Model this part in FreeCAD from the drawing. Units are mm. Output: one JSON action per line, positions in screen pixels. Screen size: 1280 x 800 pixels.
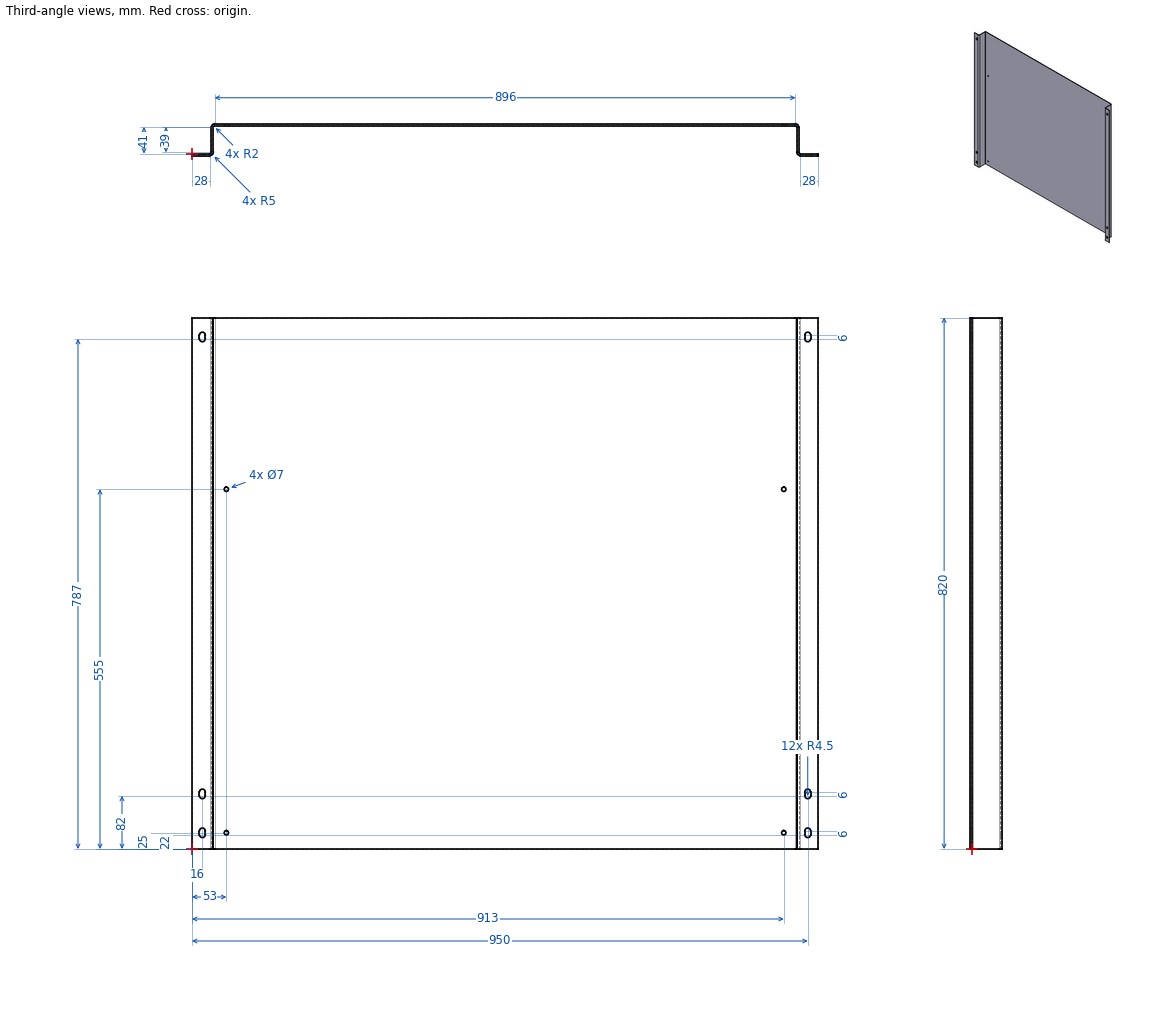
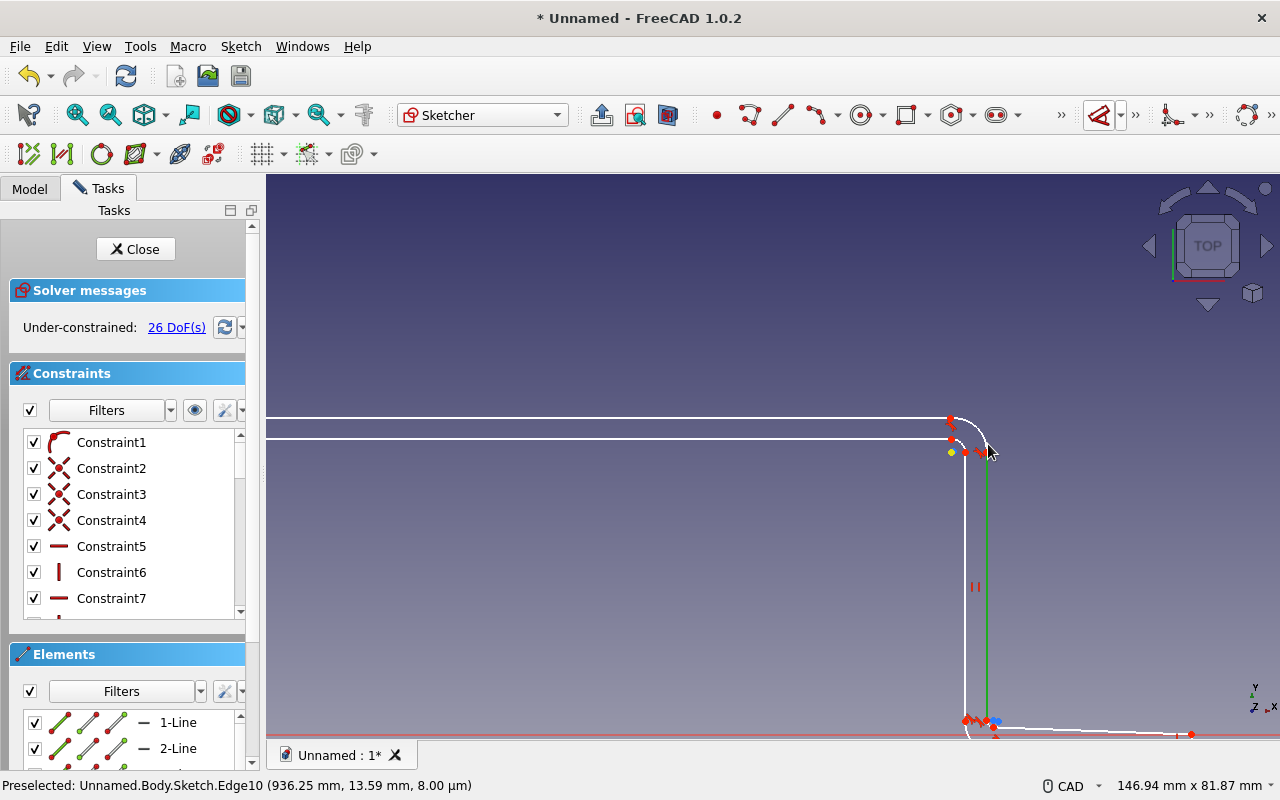
{"action": "left_click", "coordinate": [983, 436]}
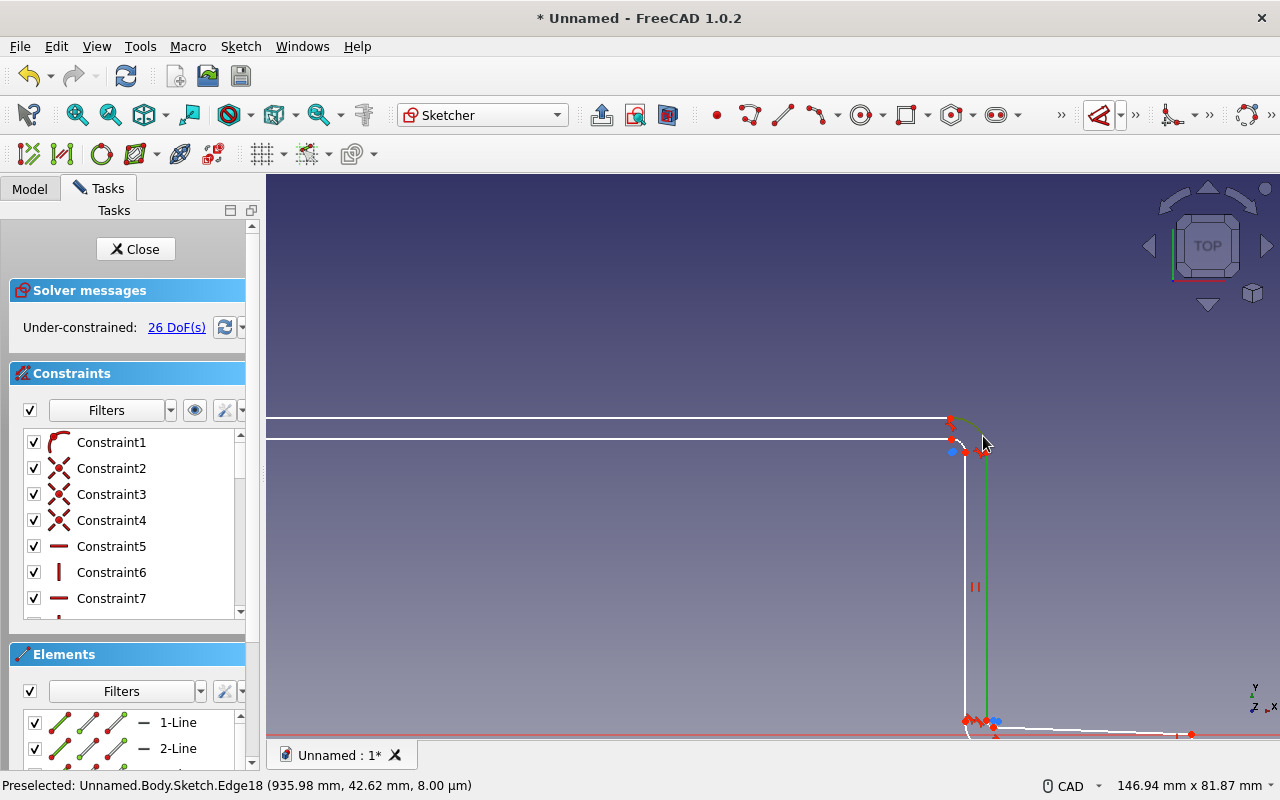
{"action": "key", "text": "t"}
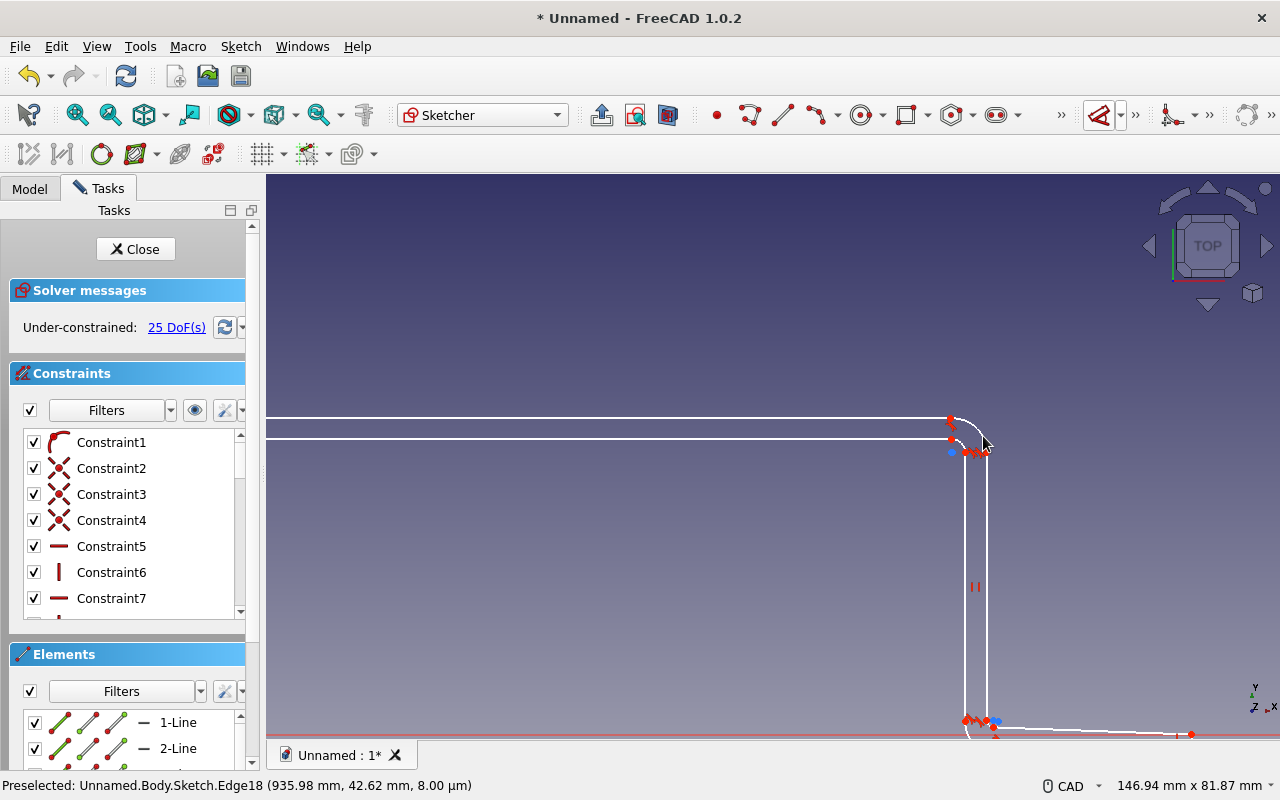
{"action": "scroll", "coordinate": [988, 444], "scroll_direction": "down", "scroll_amount": 12}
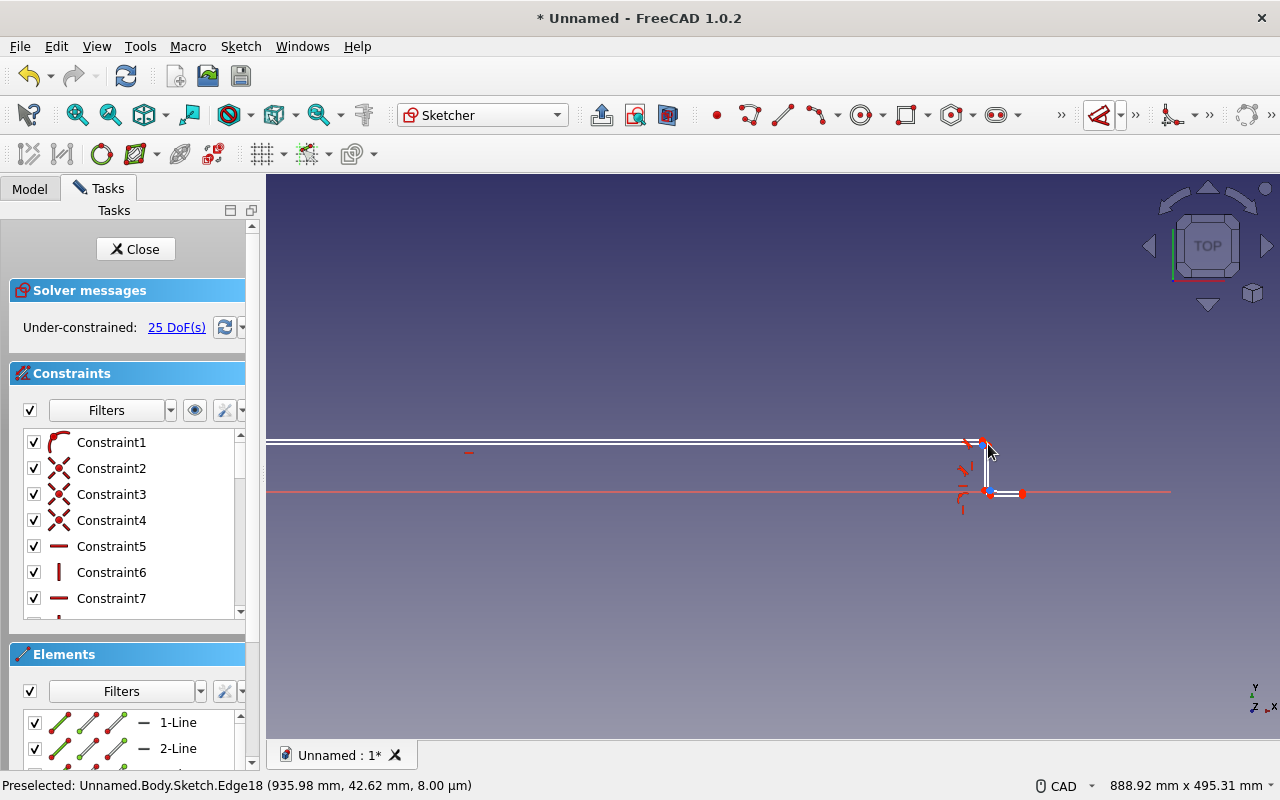
{"action": "scroll", "coordinate": [817, 442], "scroll_direction": "up", "scroll_amount": 10}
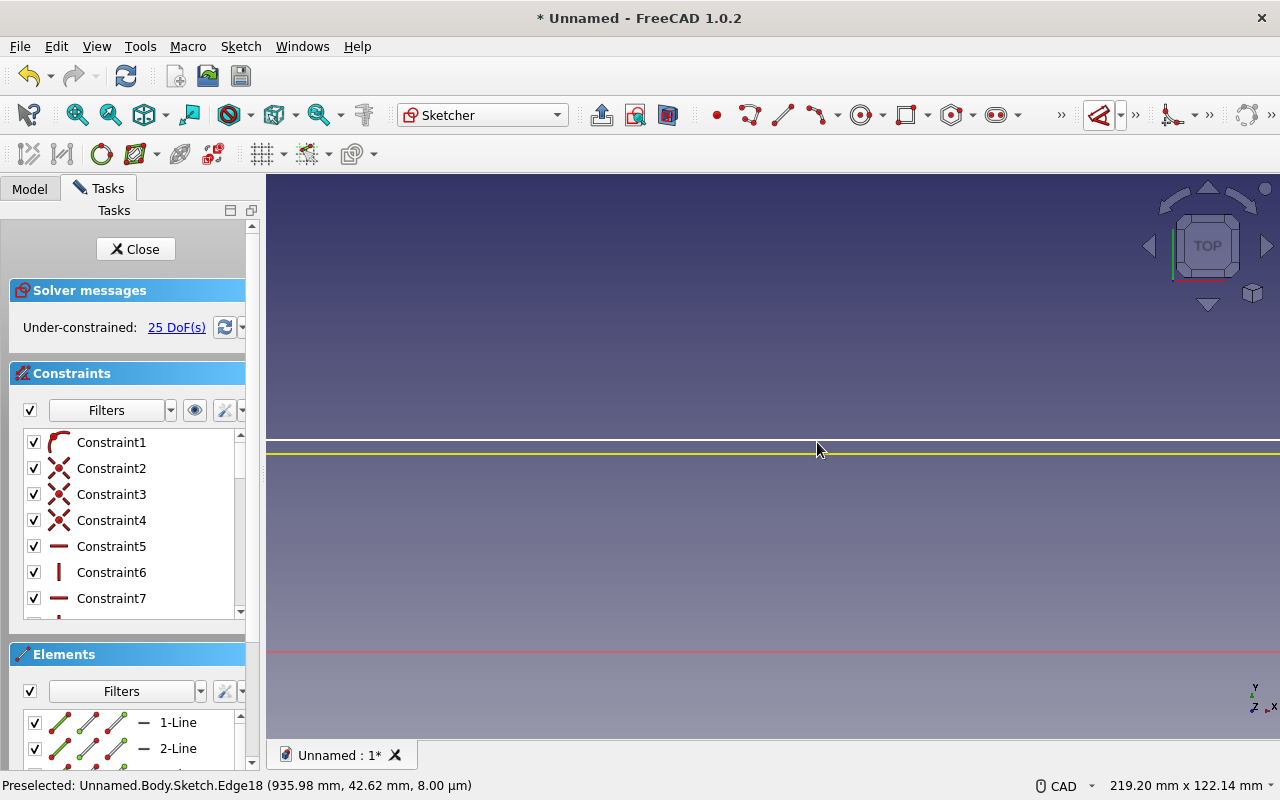
{"action": "left_click", "coordinate": [813, 440]}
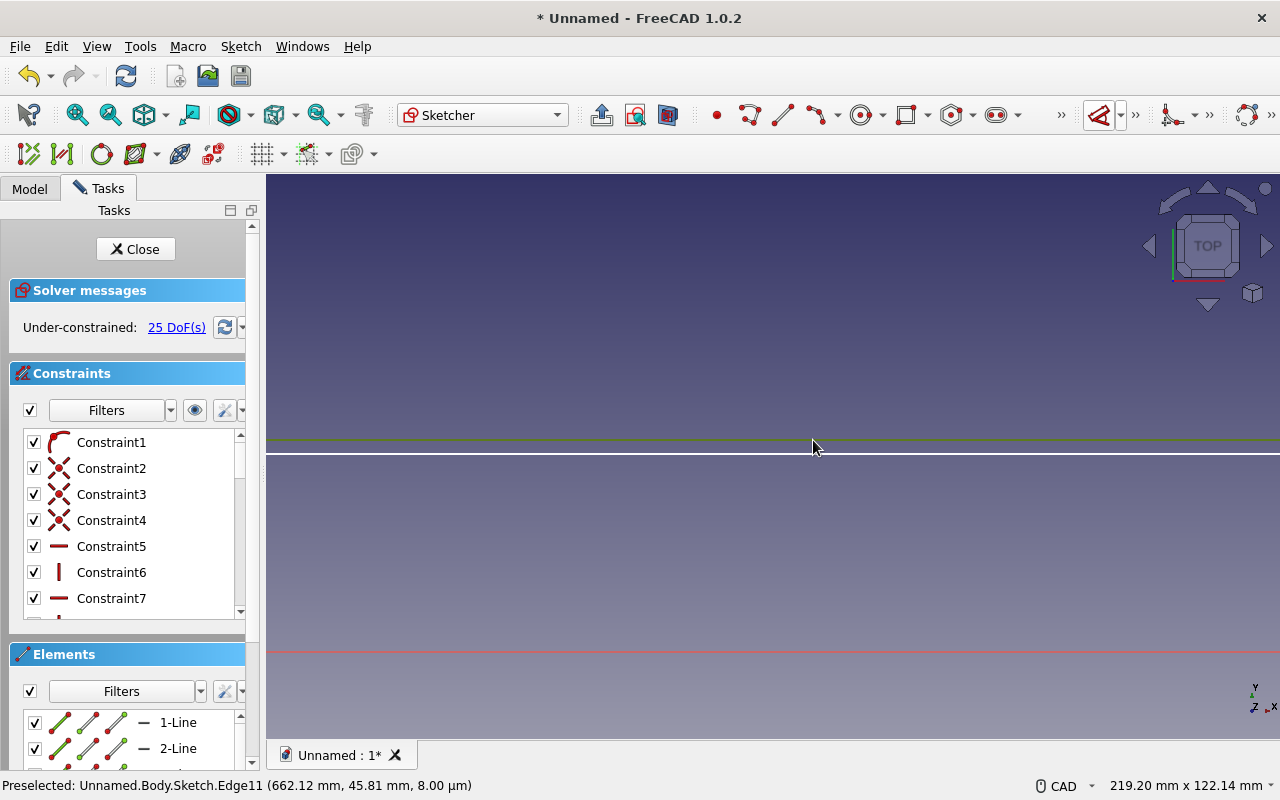
{"action": "scroll", "coordinate": [817, 442], "scroll_direction": "down", "scroll_amount": 10}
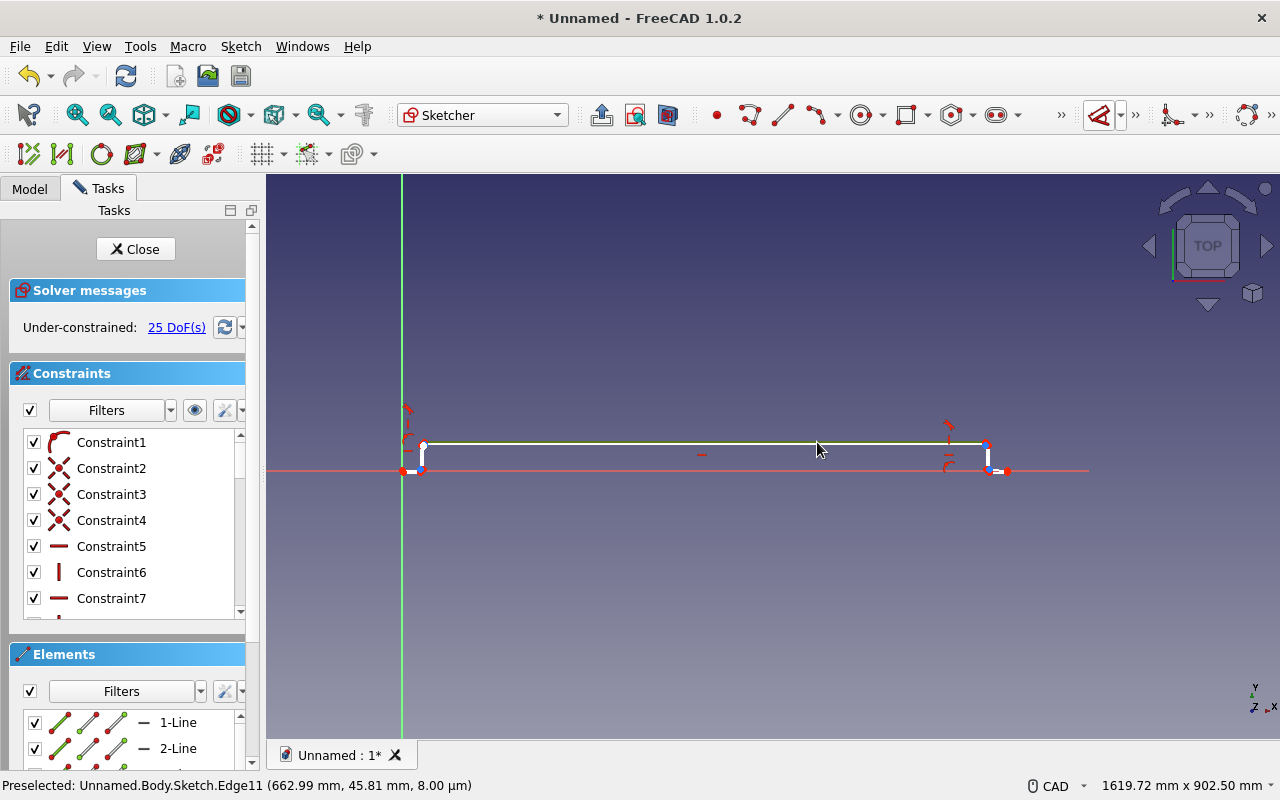
{"action": "scroll", "coordinate": [988, 444], "scroll_direction": "up", "scroll_amount": 12}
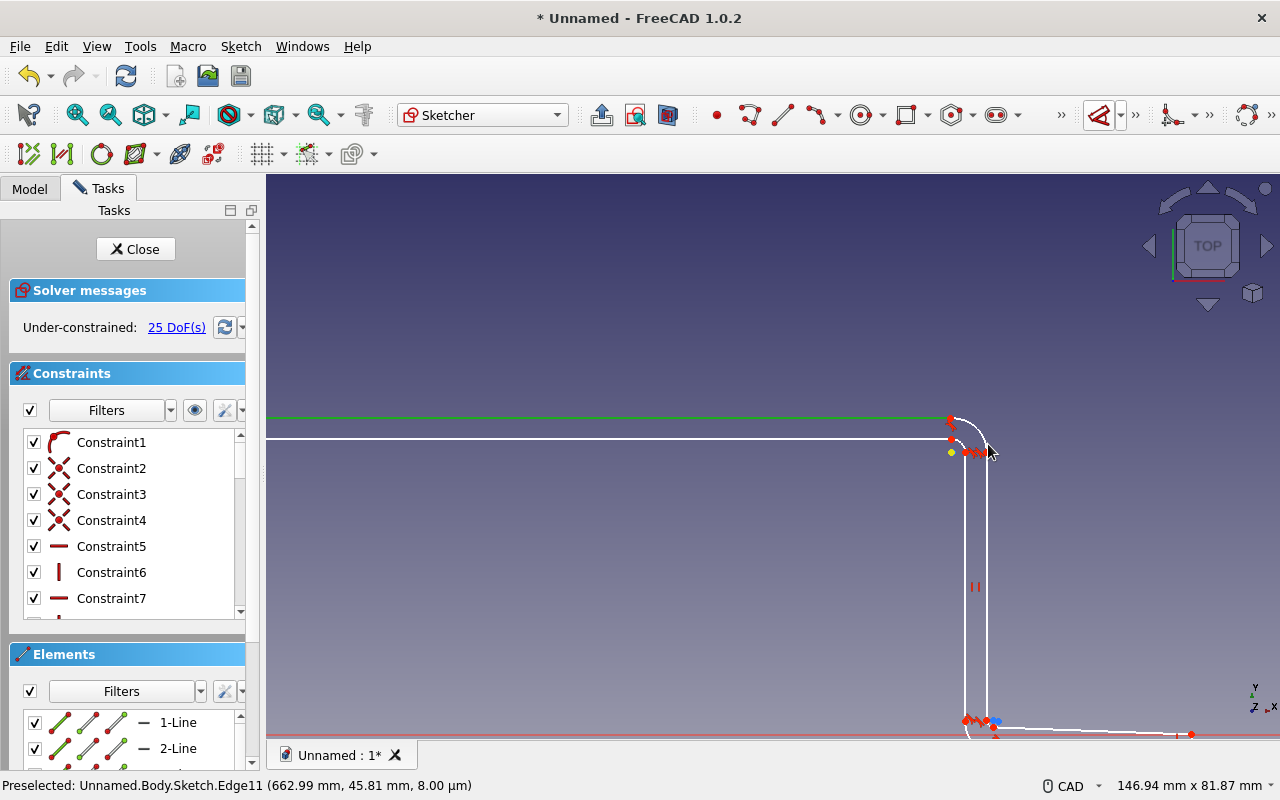
{"action": "left_click", "coordinate": [983, 436]}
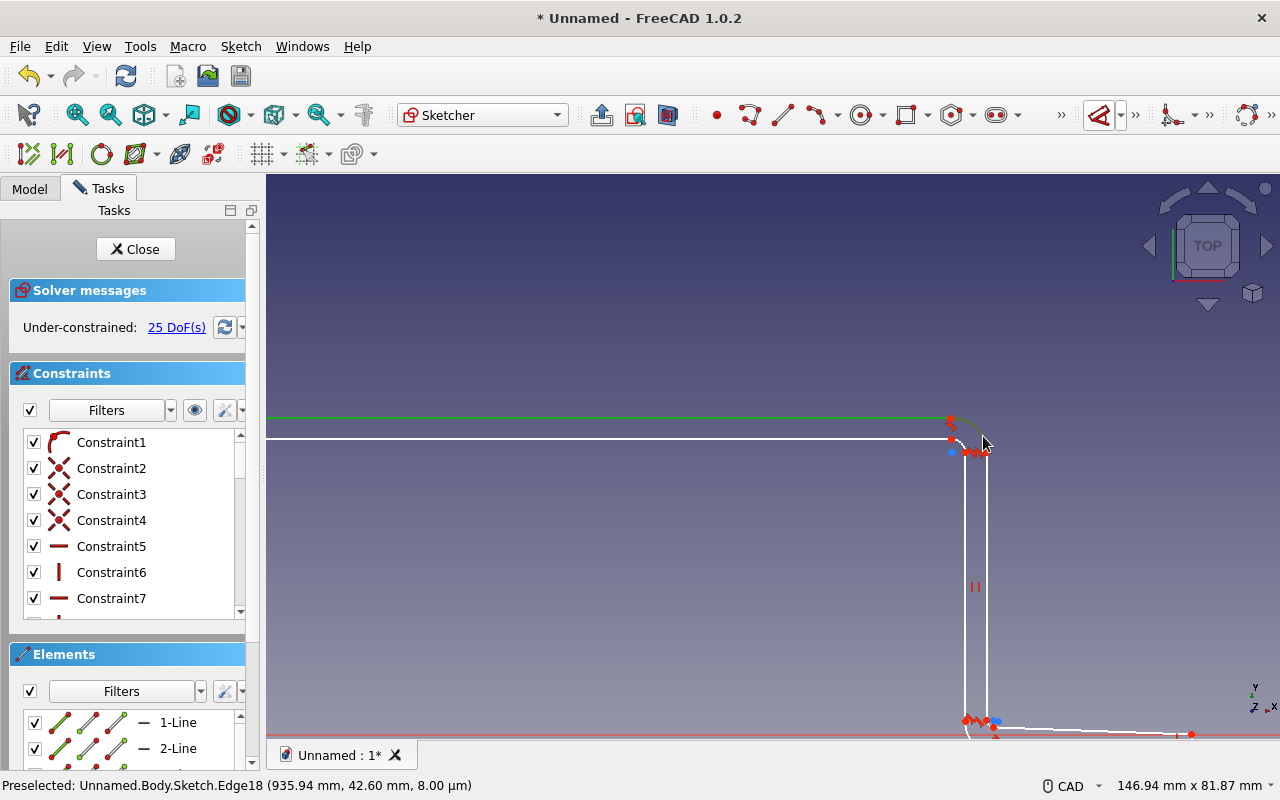
{"action": "key", "text": "t"}